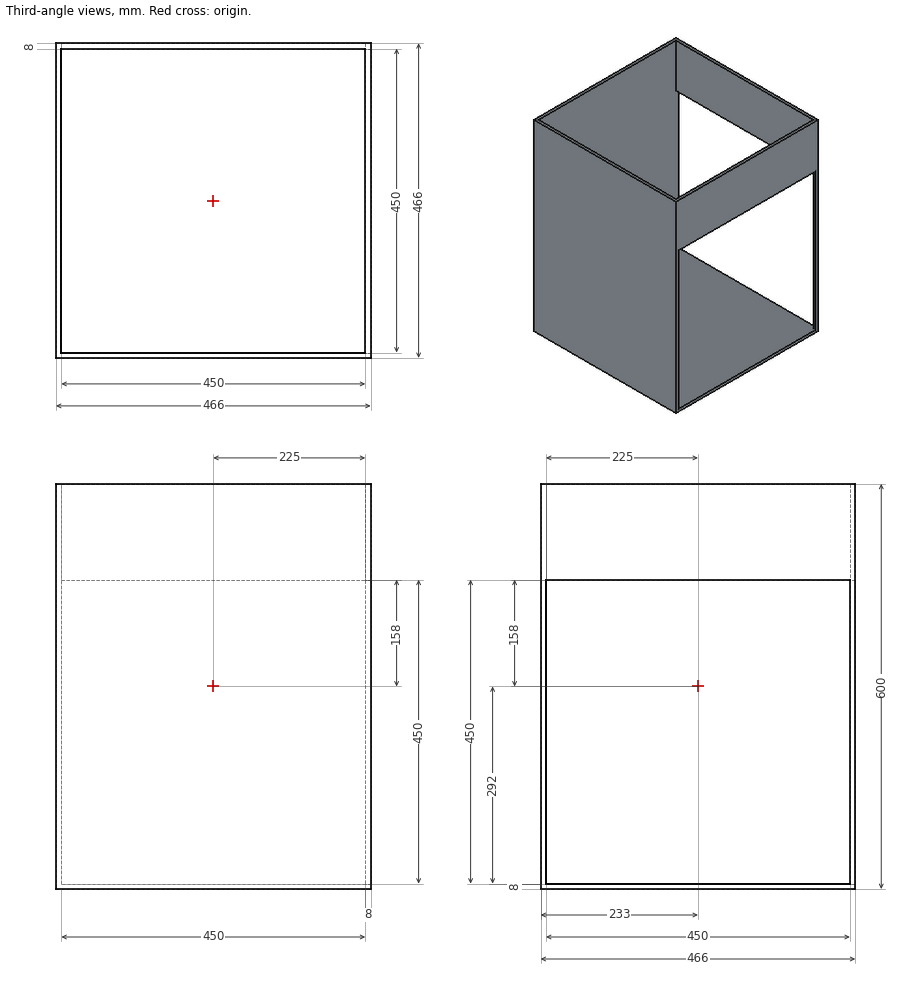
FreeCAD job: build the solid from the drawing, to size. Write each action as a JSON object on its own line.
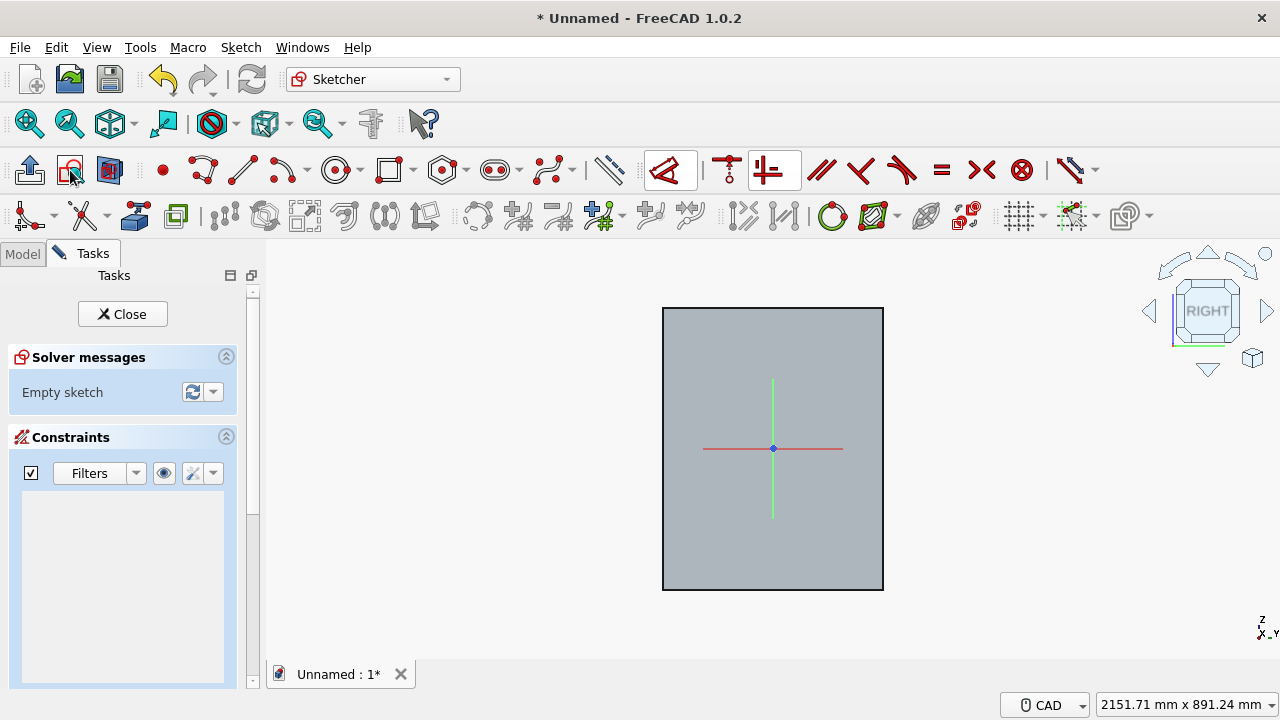
{"action": "left_click", "coordinate": [390, 170]}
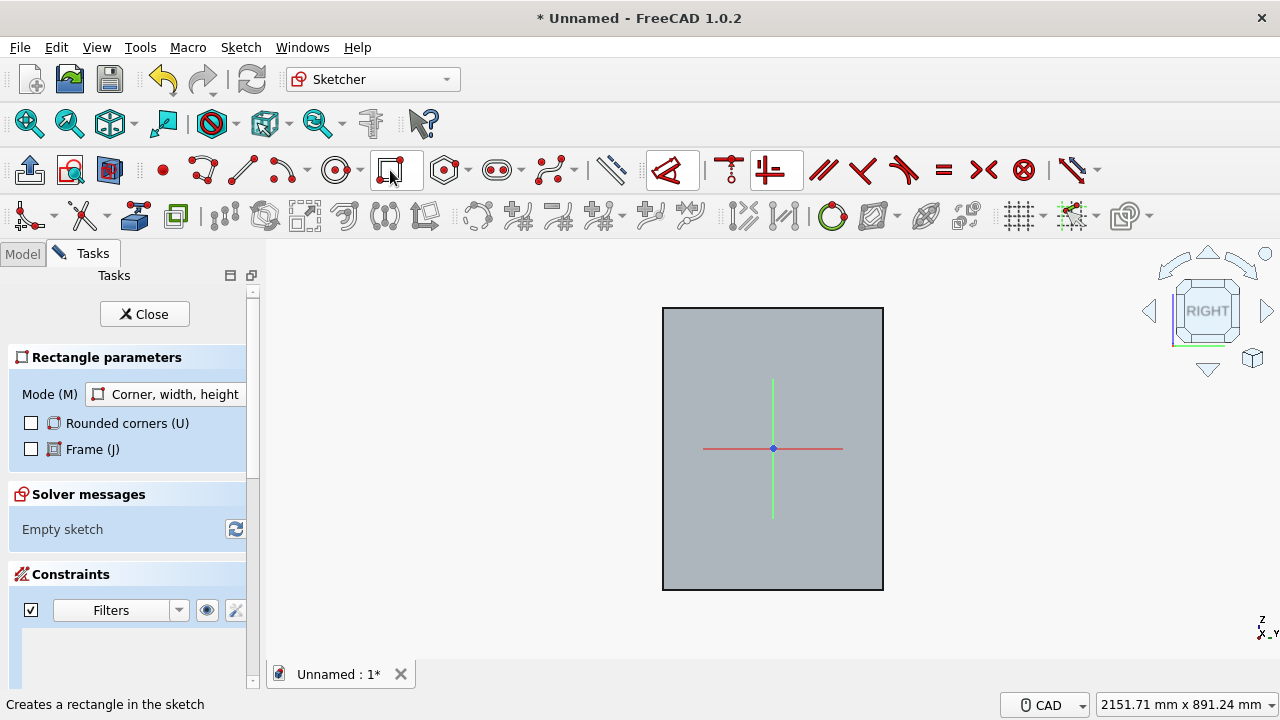
{"action": "left_click", "coordinate": [667, 375]}
{"action": "left_click", "coordinate": [879, 587]}
{"action": "key", "text": "Escape"}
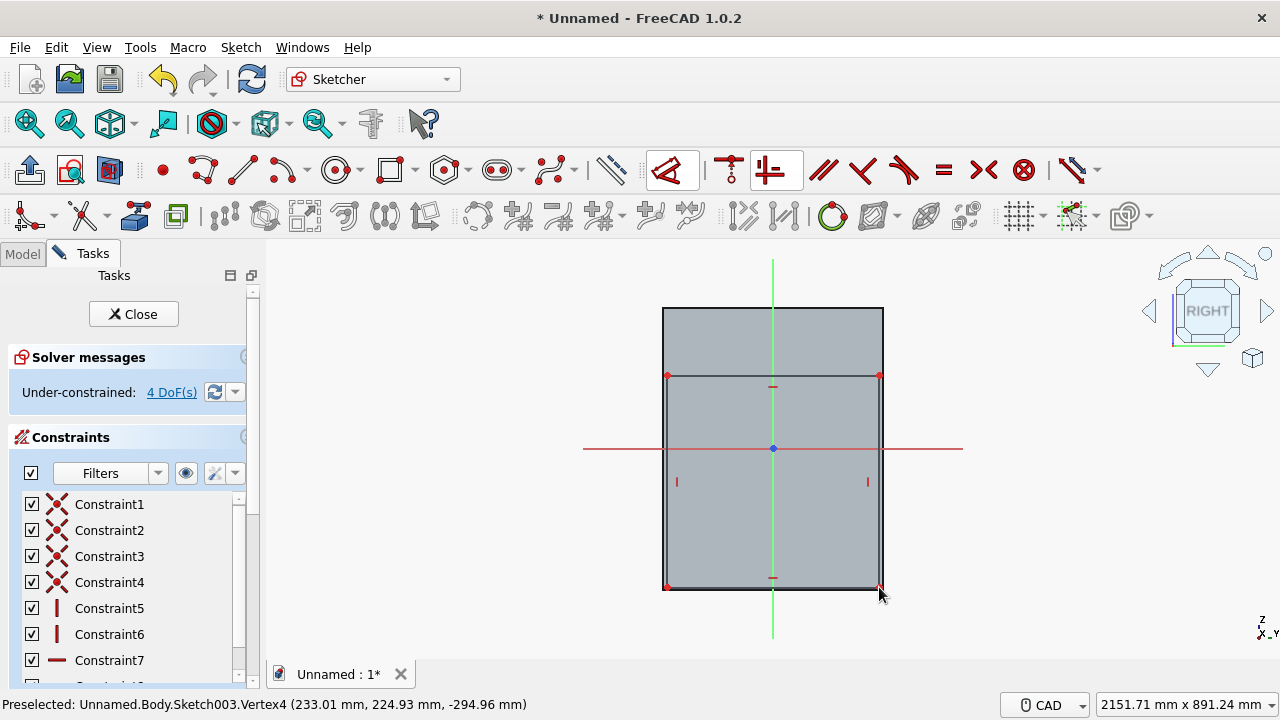
{"action": "scroll", "coordinate": [667, 440], "scroll_direction": "up", "scroll_amount": 2}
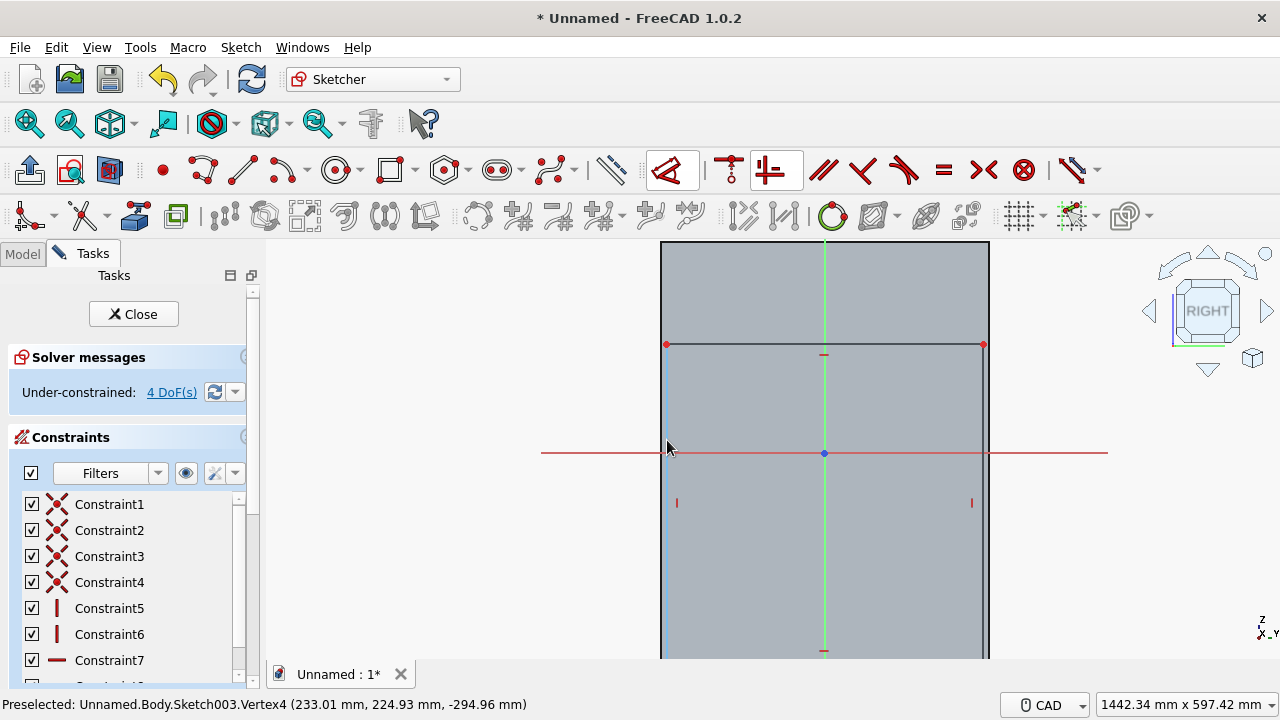
{"action": "left_click", "coordinate": [667, 439]}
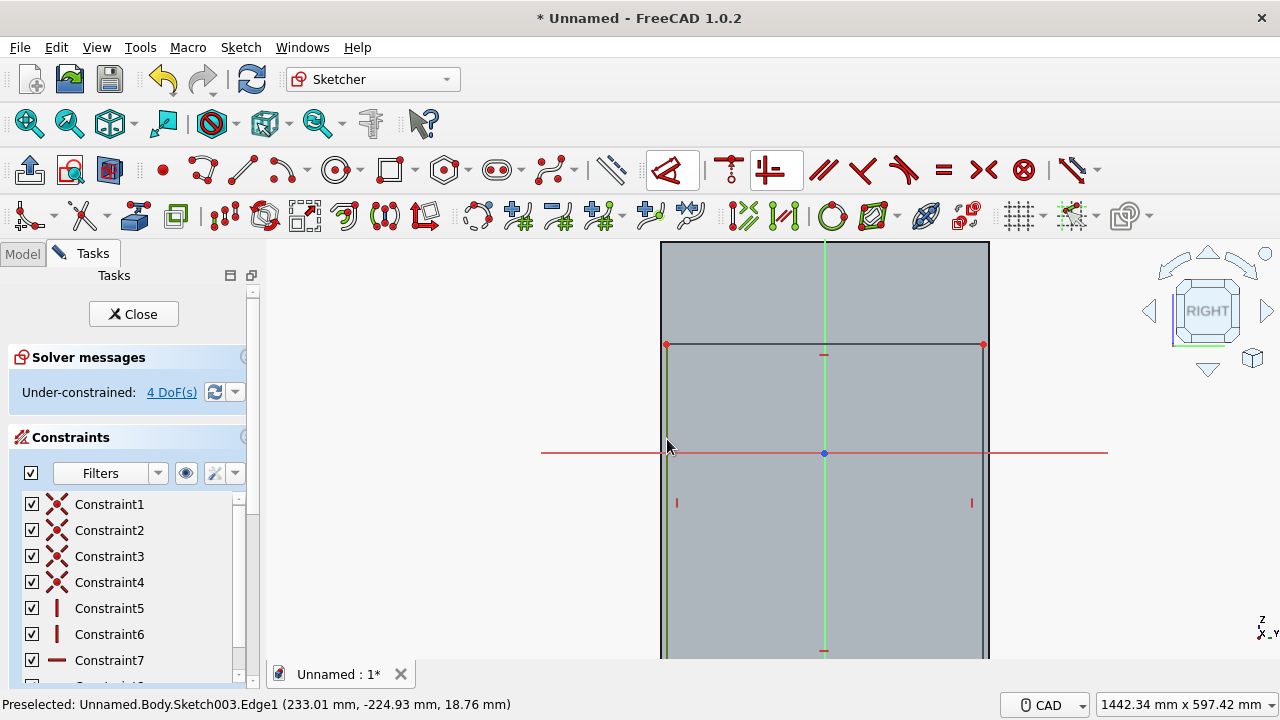
{"action": "key", "text": "i"}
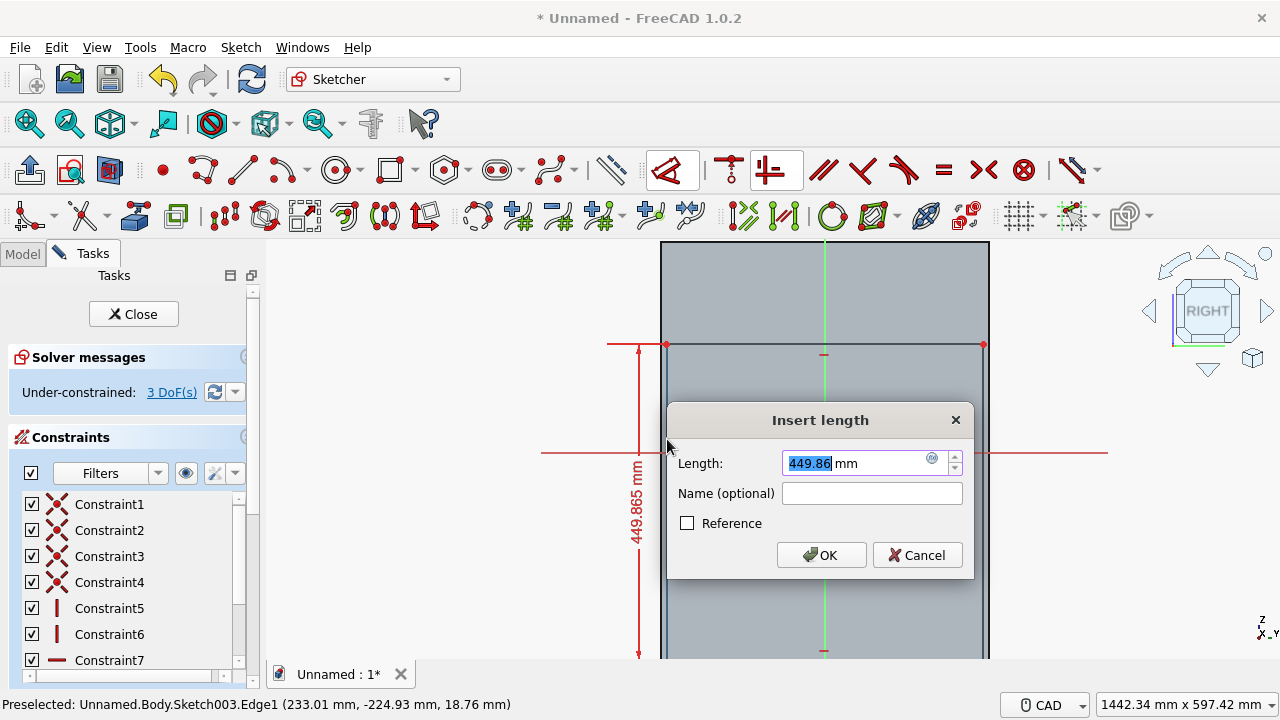
{"action": "type", "text": "450"}
{"action": "key", "text": "Return"}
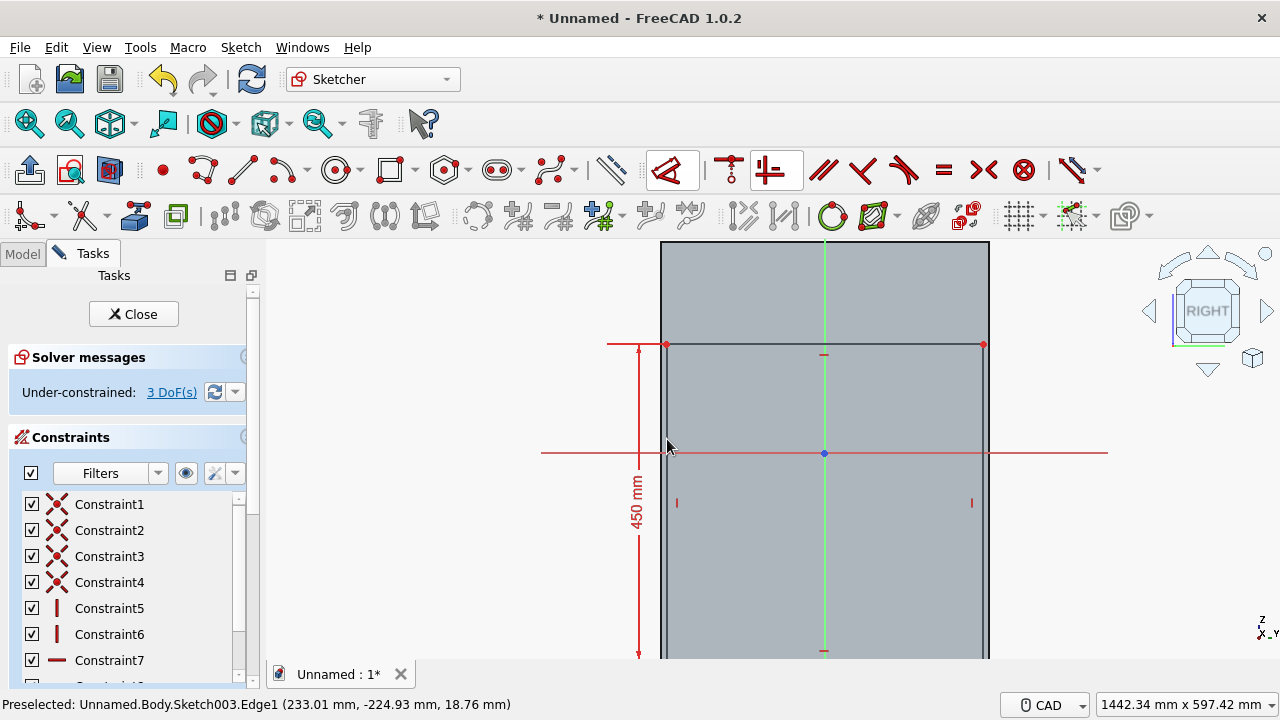
{"action": "scroll", "coordinate": [294, 267], "scroll_direction": "down", "scroll_amount": 1}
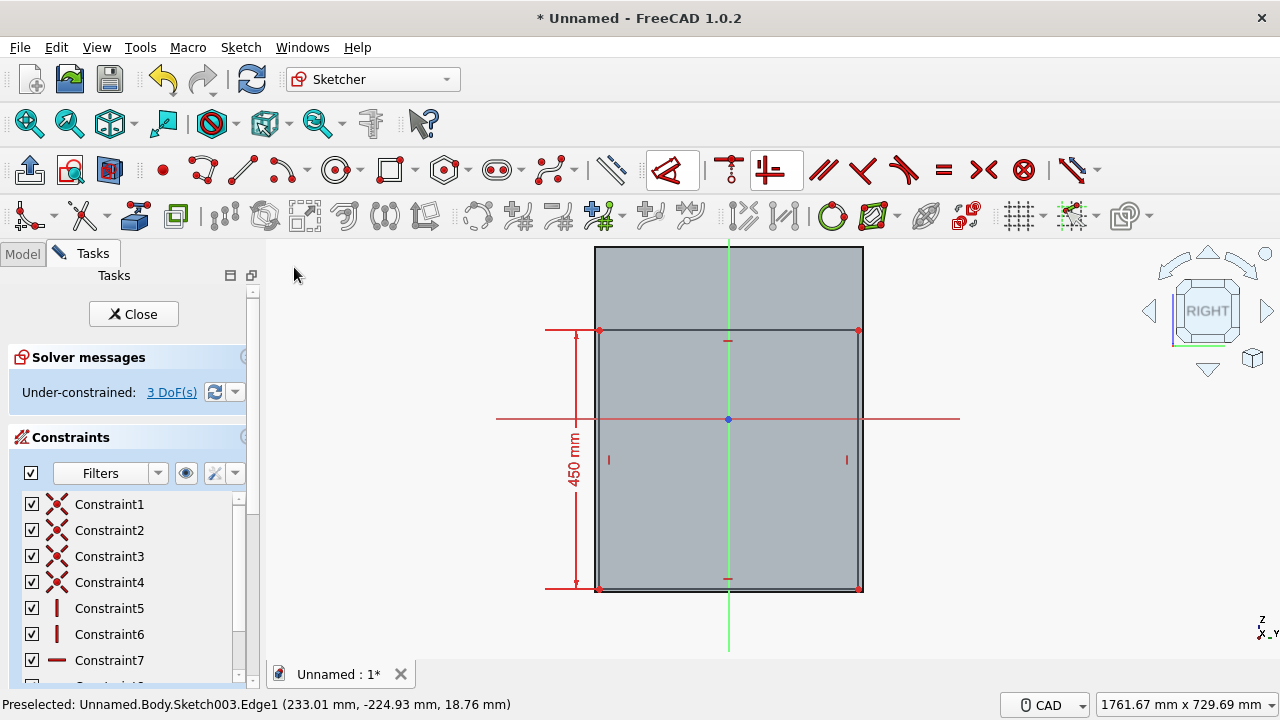
{"action": "left_click", "coordinate": [677, 589]}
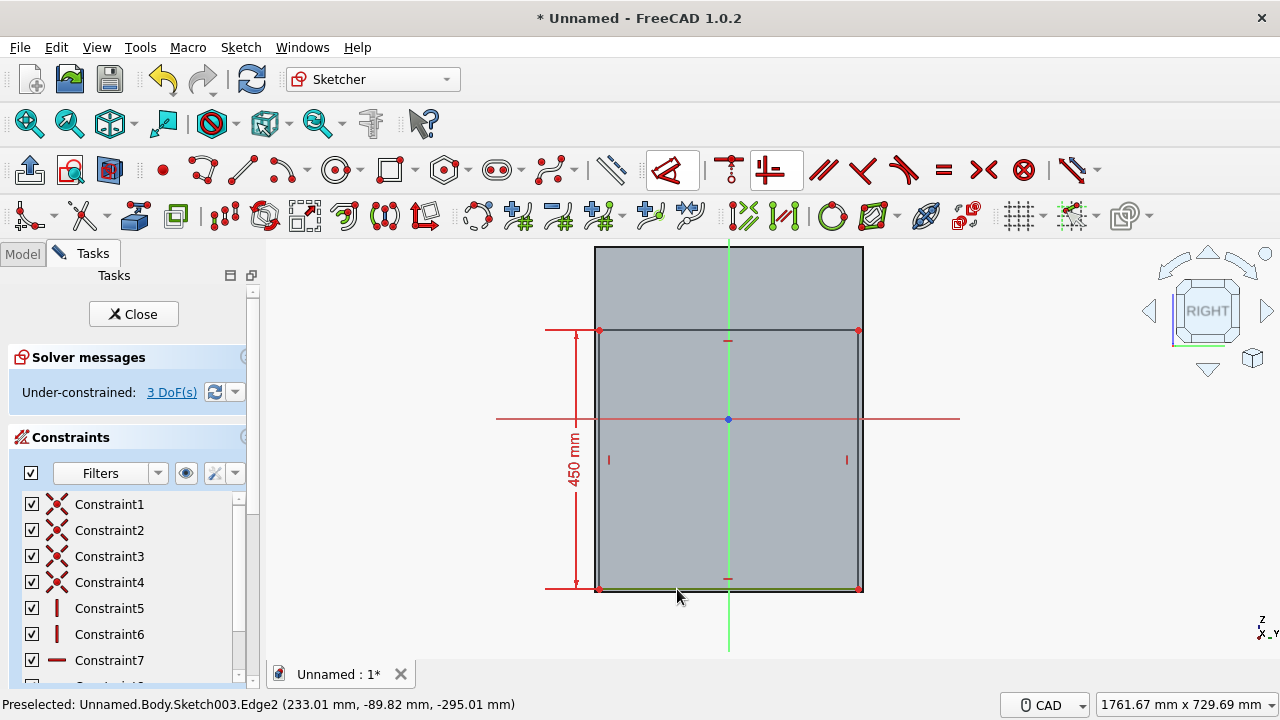
{"action": "left_click", "coordinate": [694, 170]}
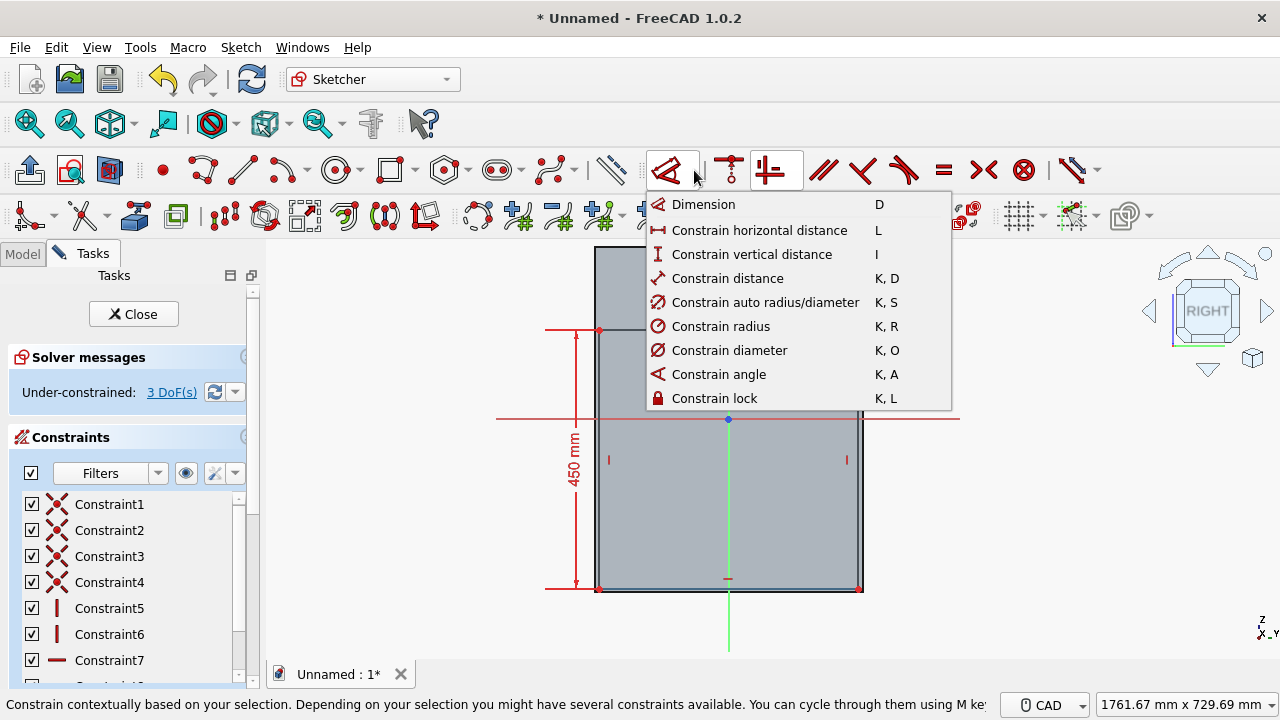
{"action": "left_click", "coordinate": [799, 230]}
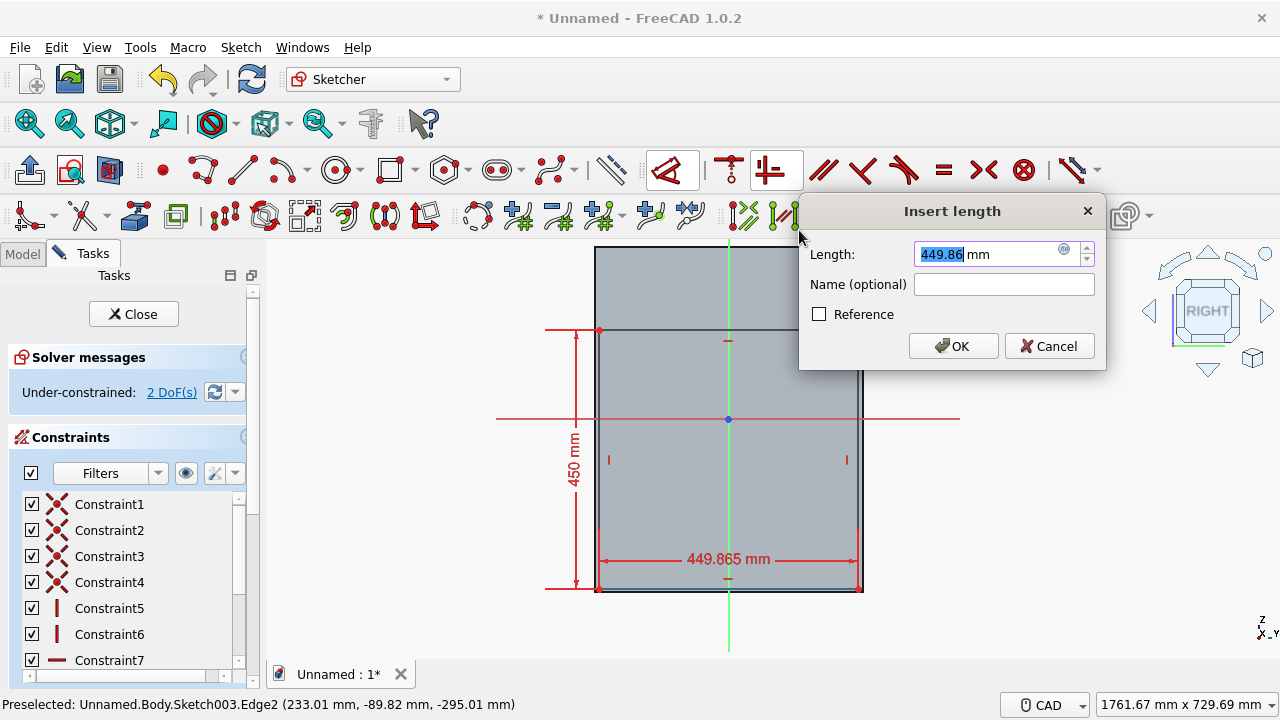
{"action": "type", "text": "450"}
{"action": "key", "text": "Return"}